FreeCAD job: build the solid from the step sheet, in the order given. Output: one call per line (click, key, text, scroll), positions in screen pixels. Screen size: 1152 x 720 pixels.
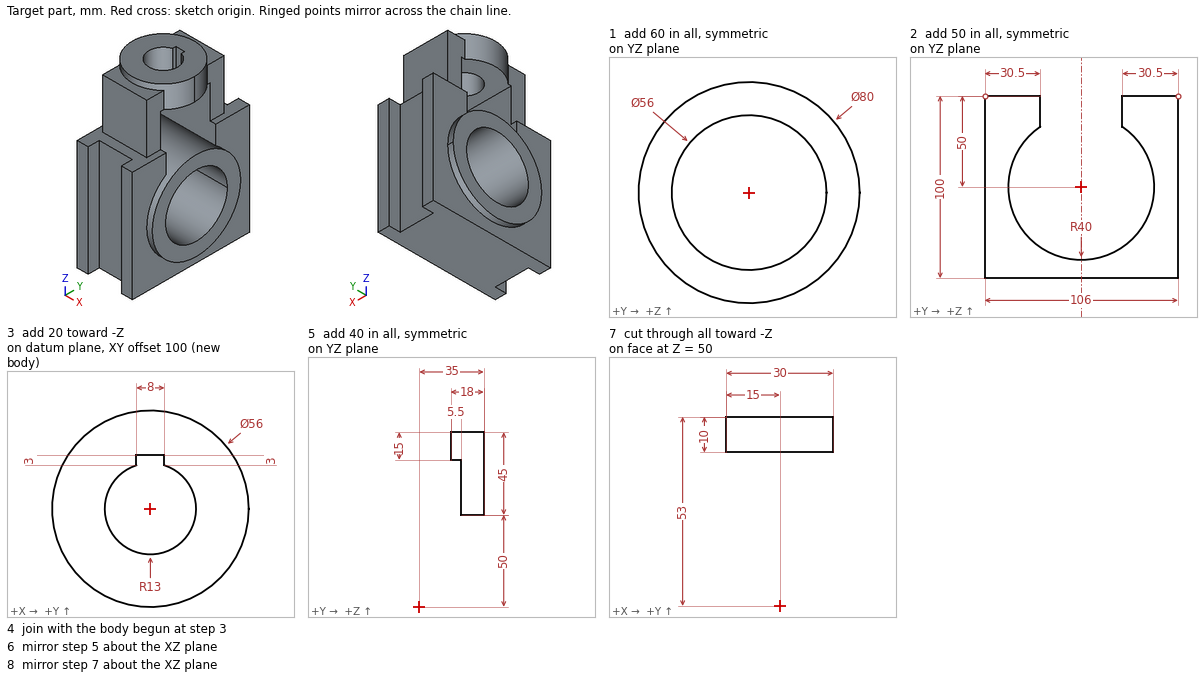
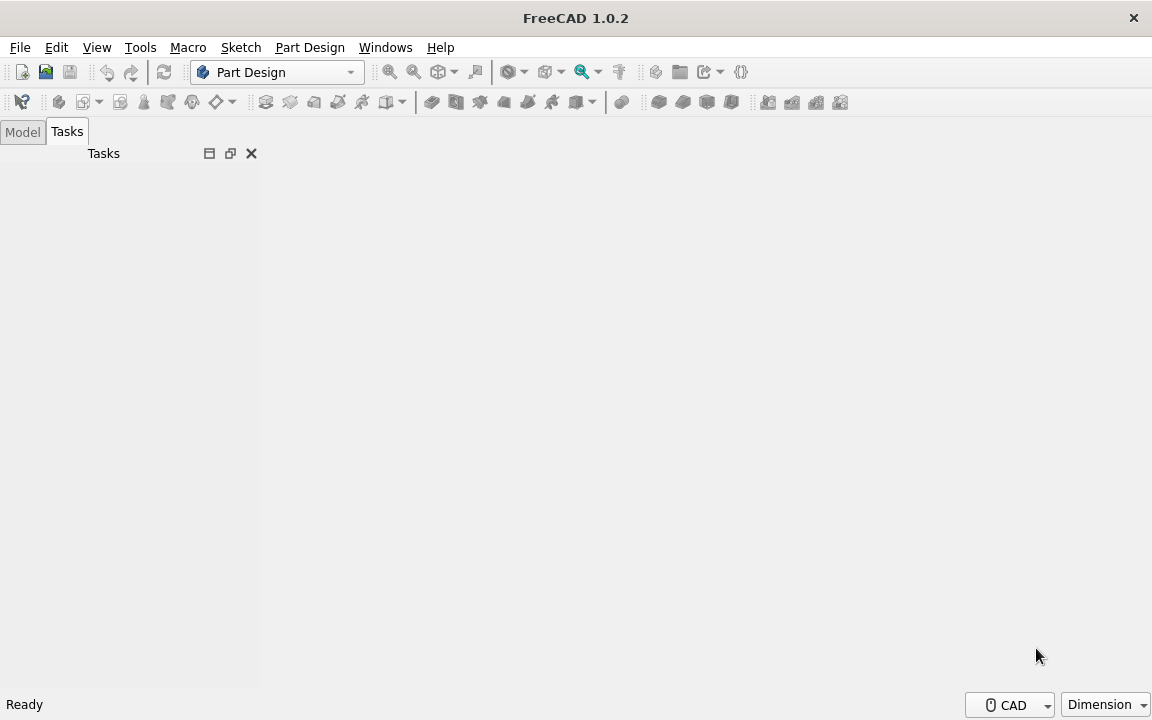
click(22, 72)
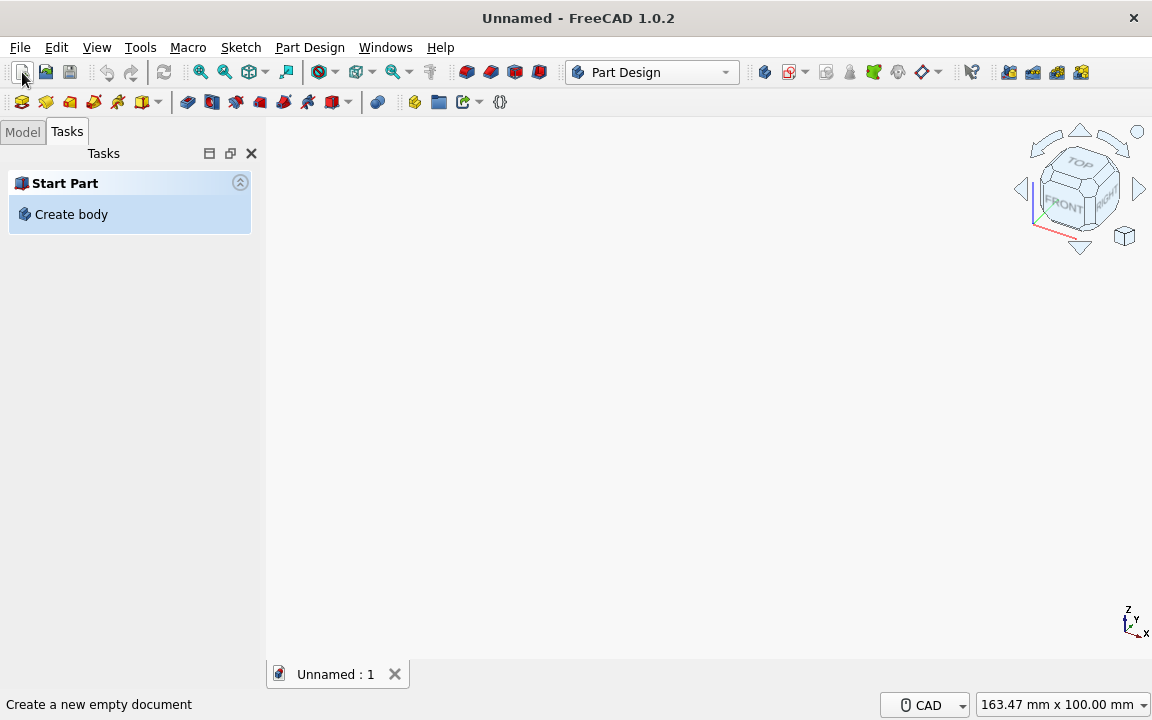
click(790, 72)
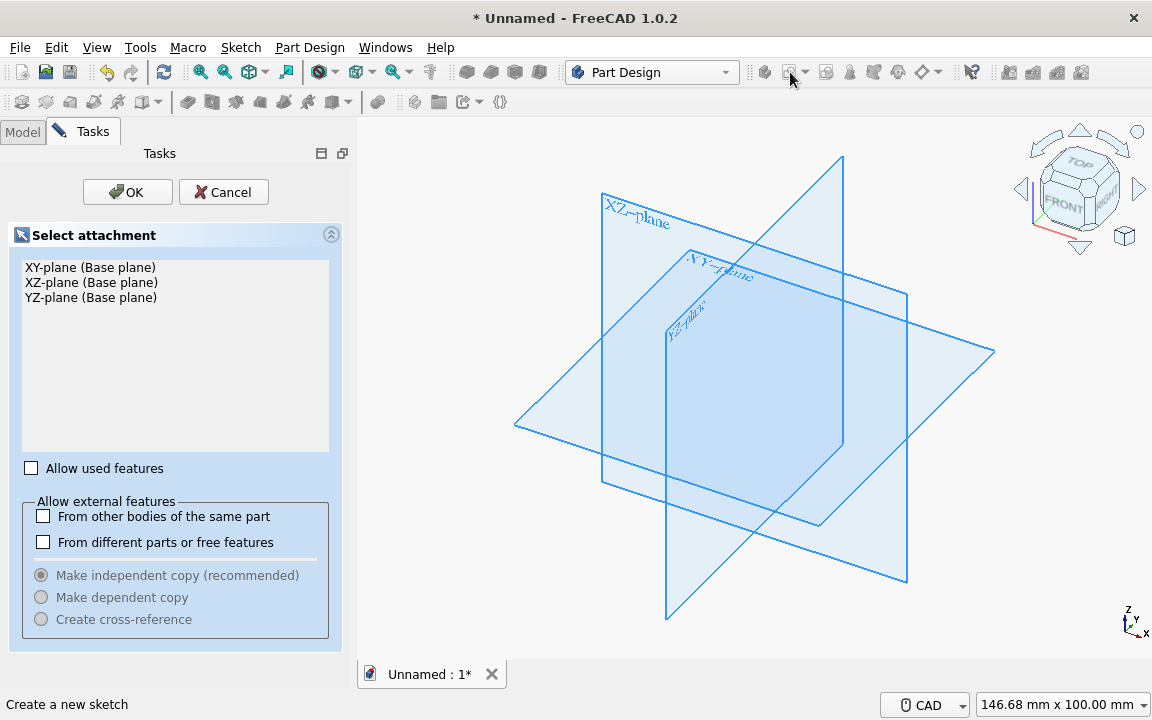
click(82, 298)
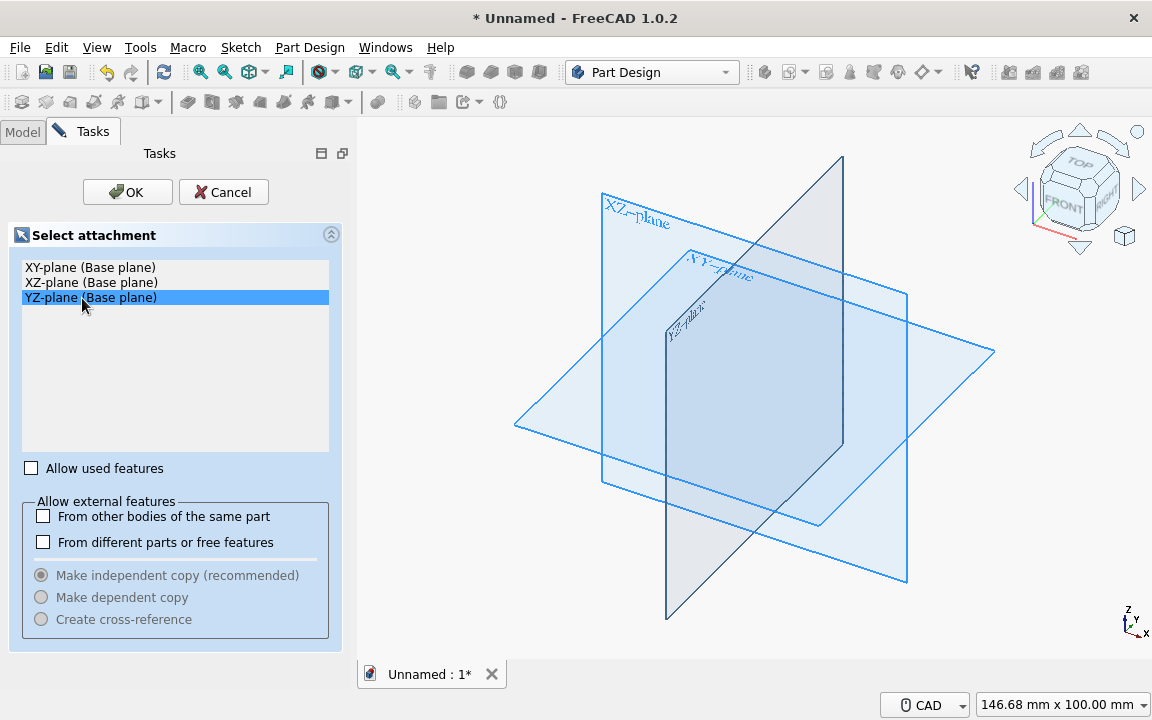
click(128, 192)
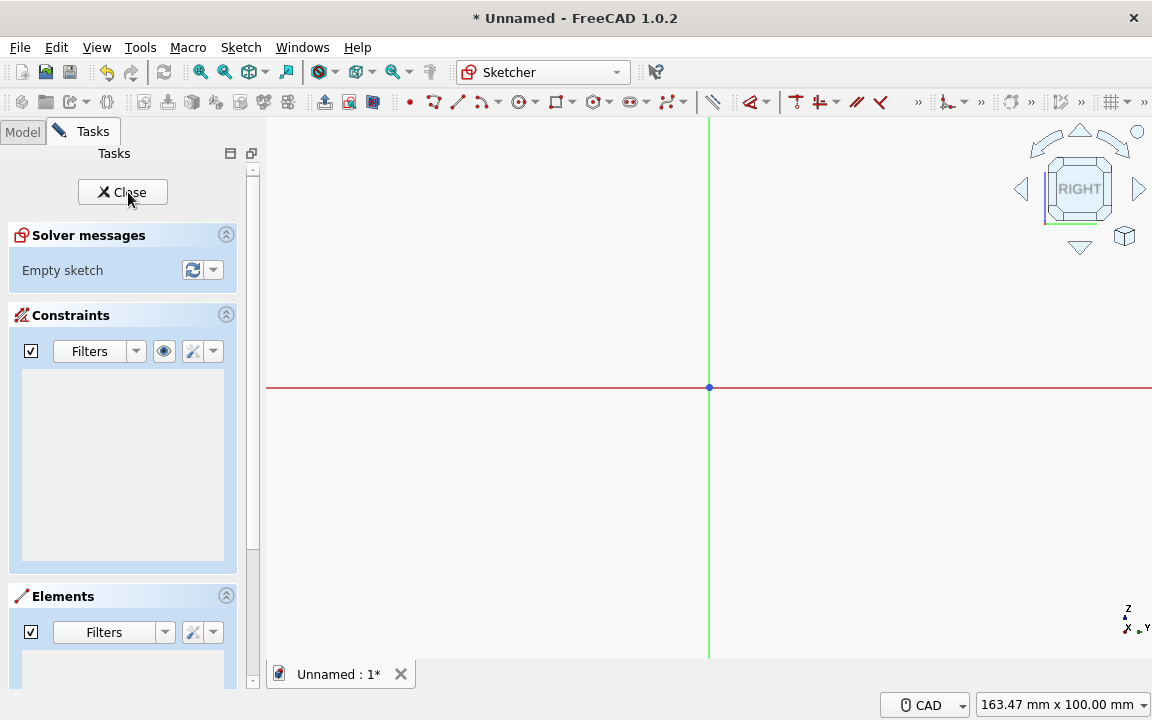
click(520, 102)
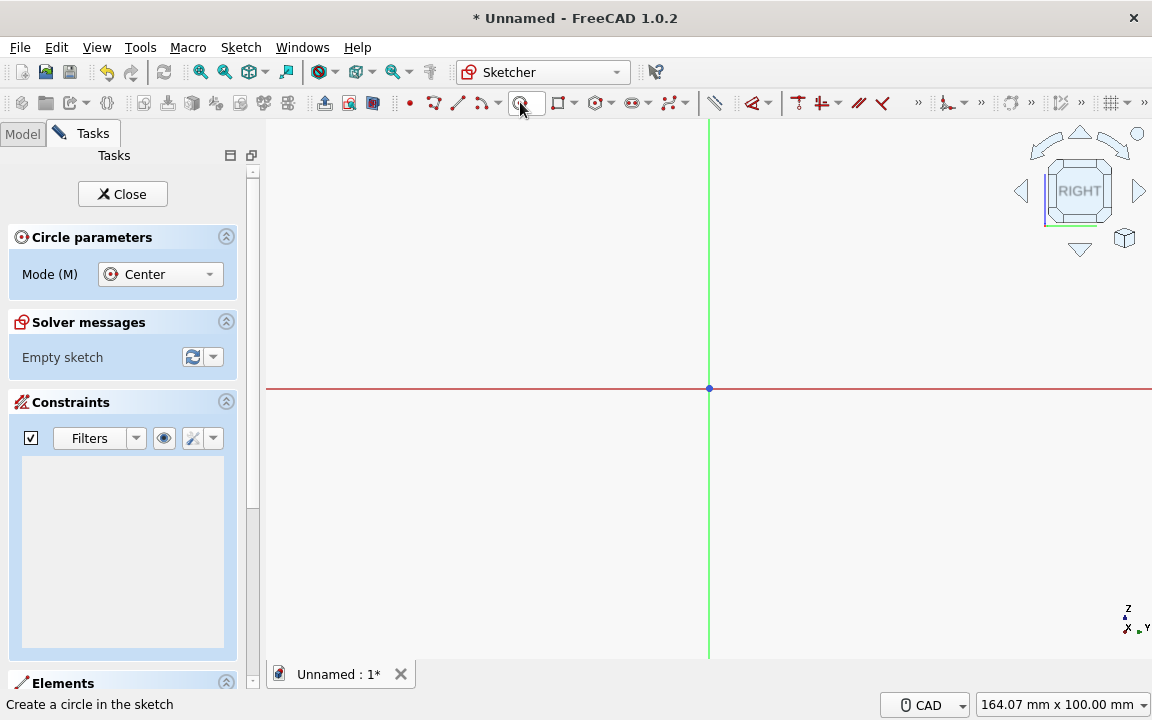
click(709, 389)
click(862, 236)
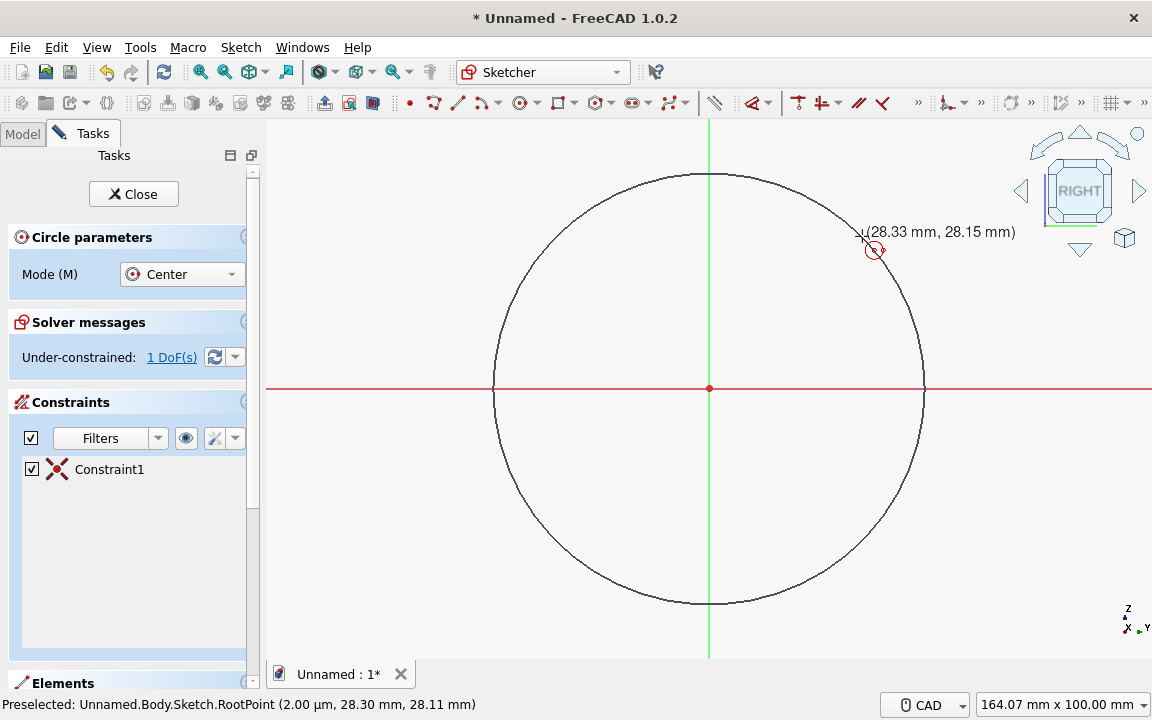
click(709, 389)
click(816, 282)
key(Escape)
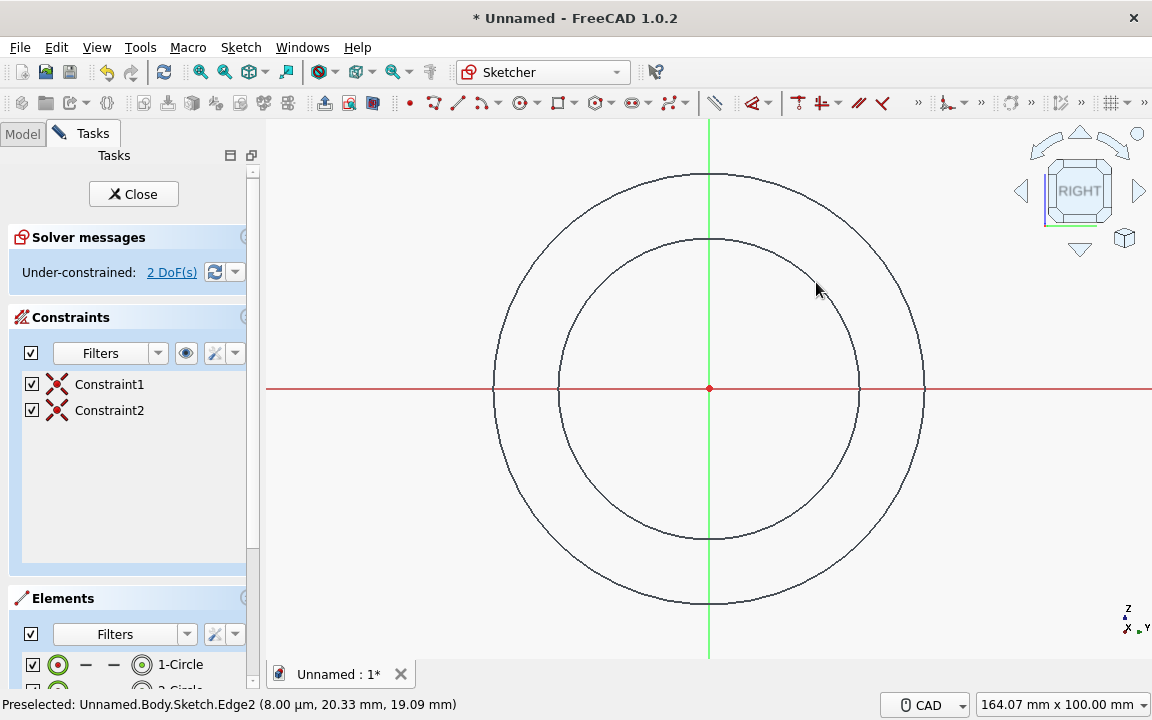
click(752, 104)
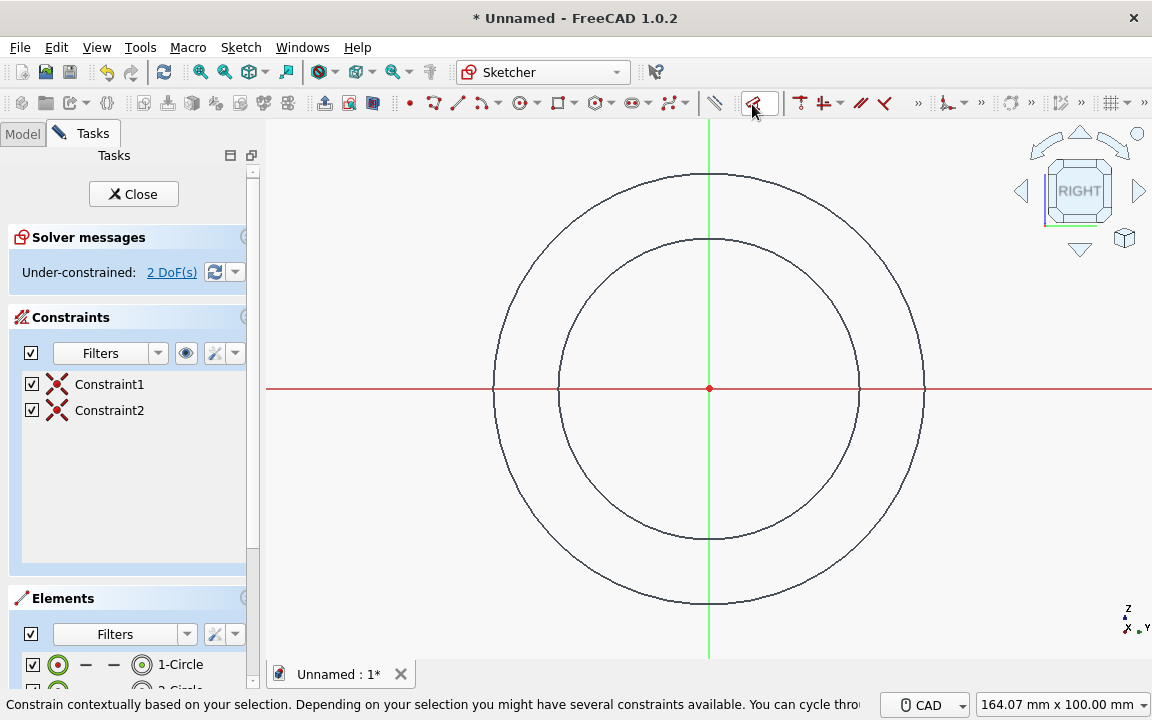
click(861, 236)
click(884, 213)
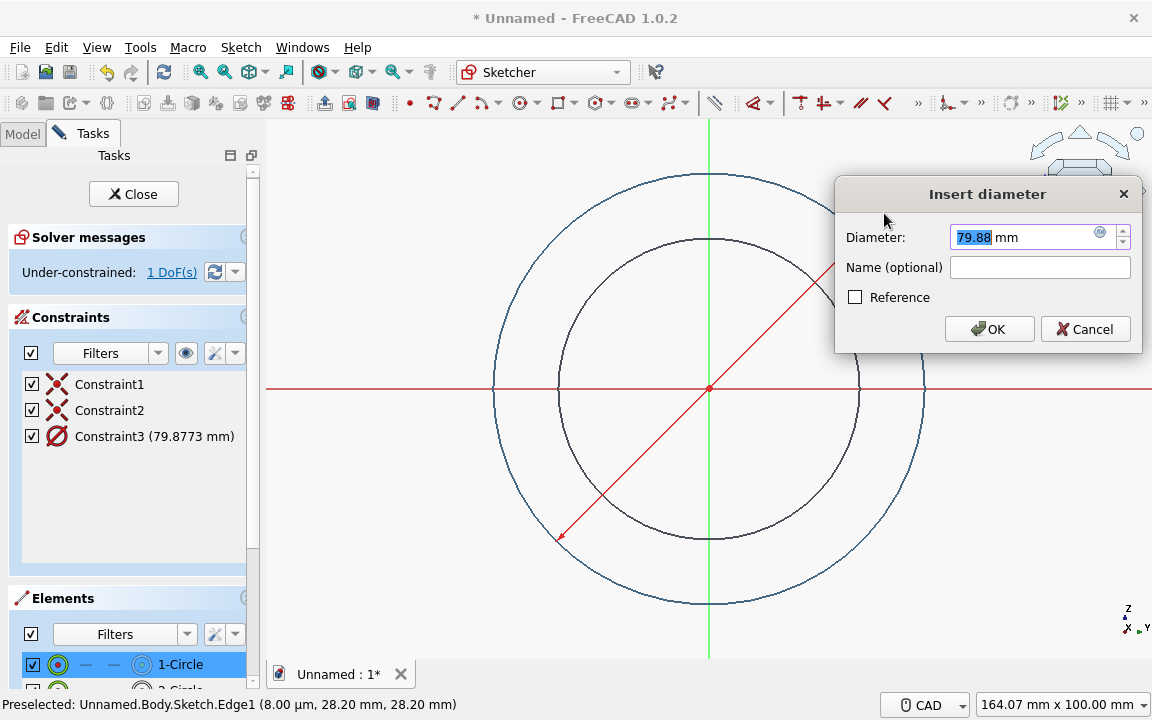
text(80)
key(Return)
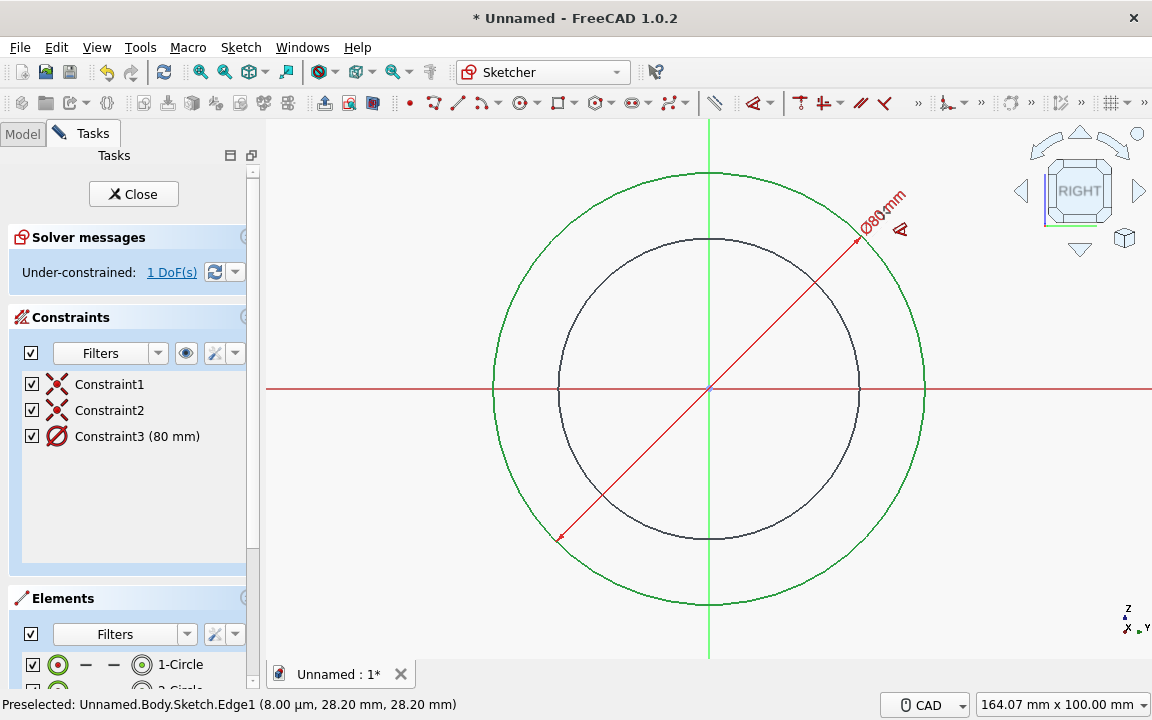
click(815, 282)
click(838, 259)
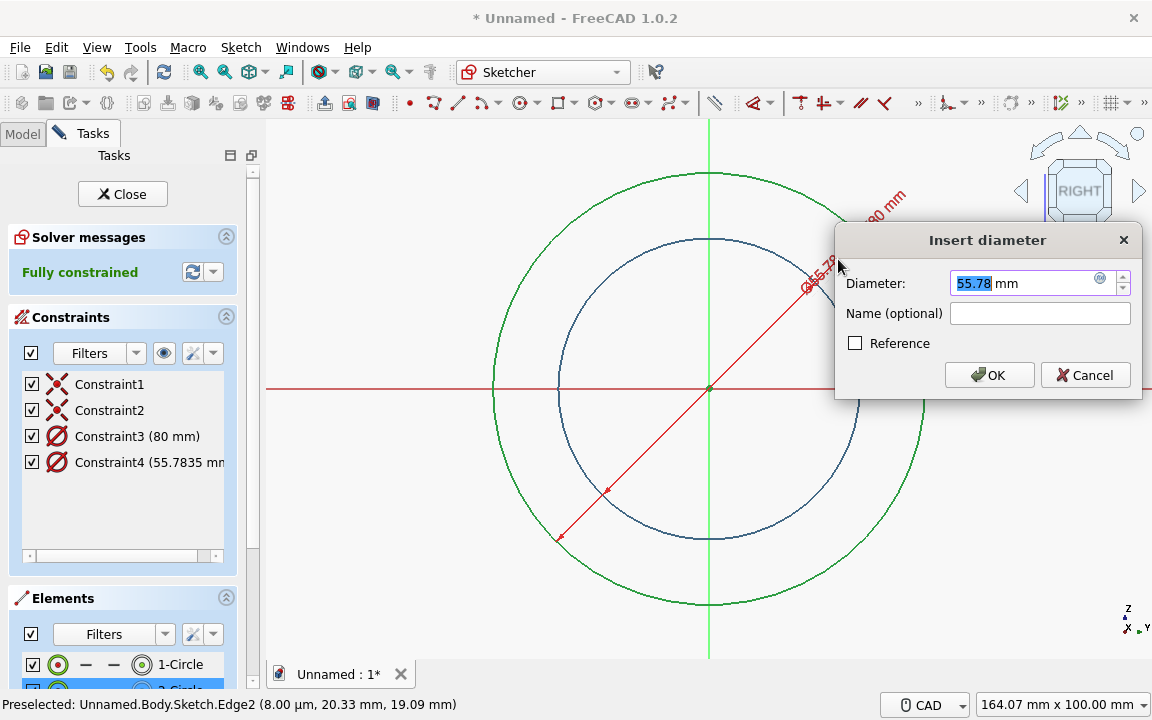
text(56)
key(Return)
key(Escape)